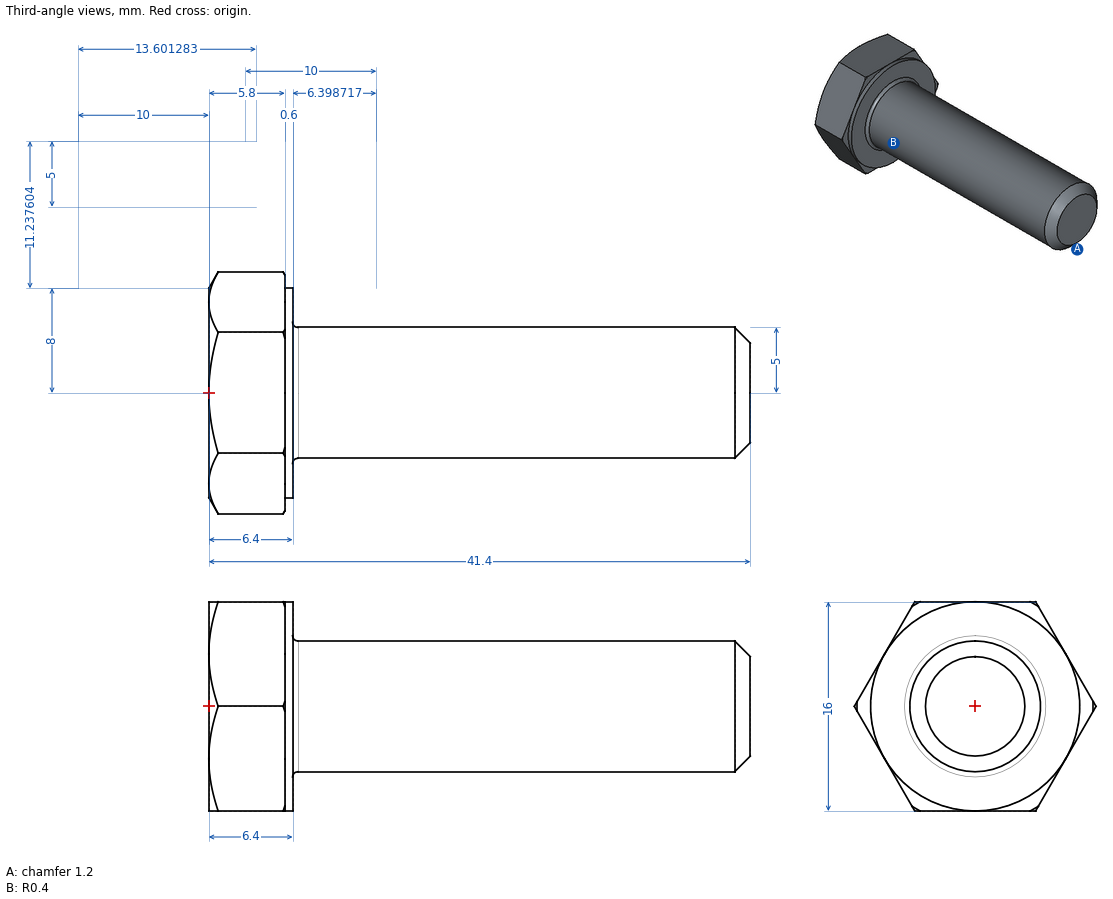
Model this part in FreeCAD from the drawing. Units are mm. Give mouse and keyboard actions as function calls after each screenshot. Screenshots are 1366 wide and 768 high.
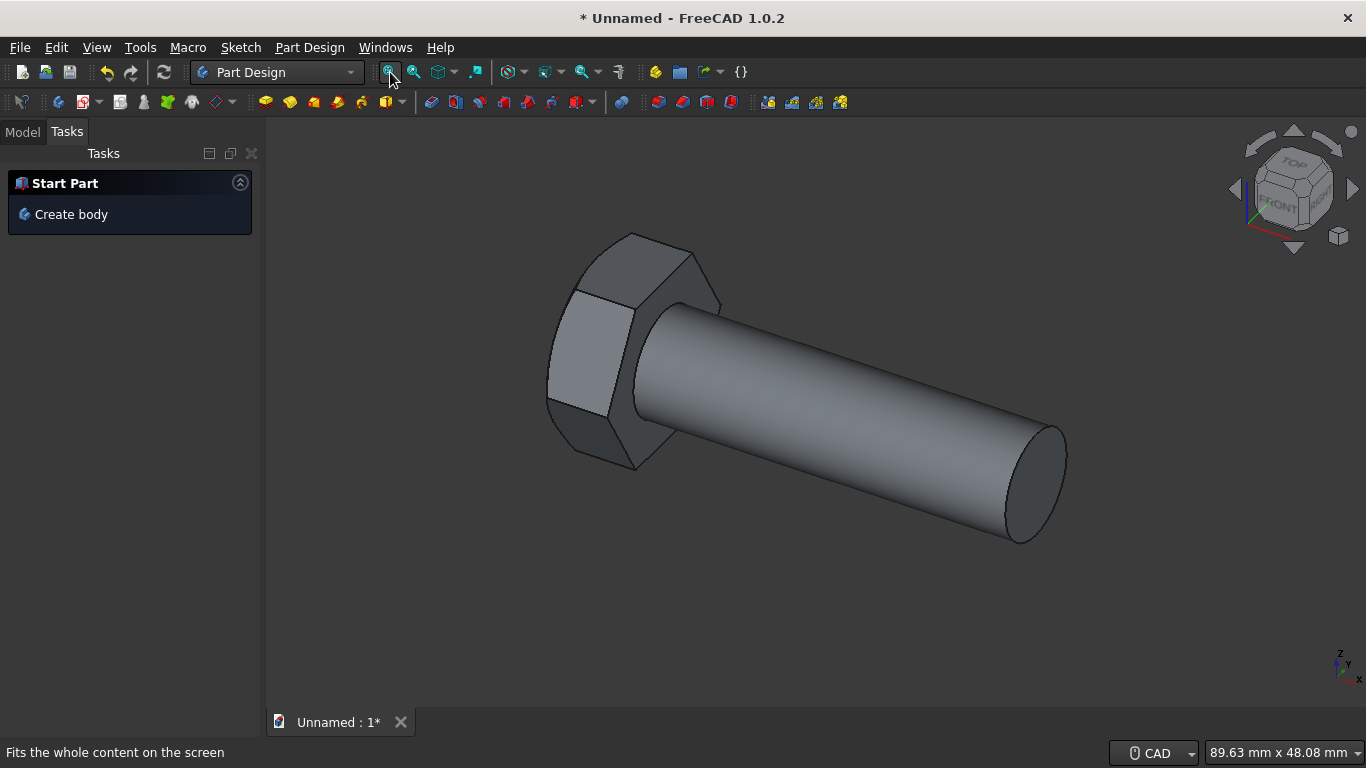
click(84, 102)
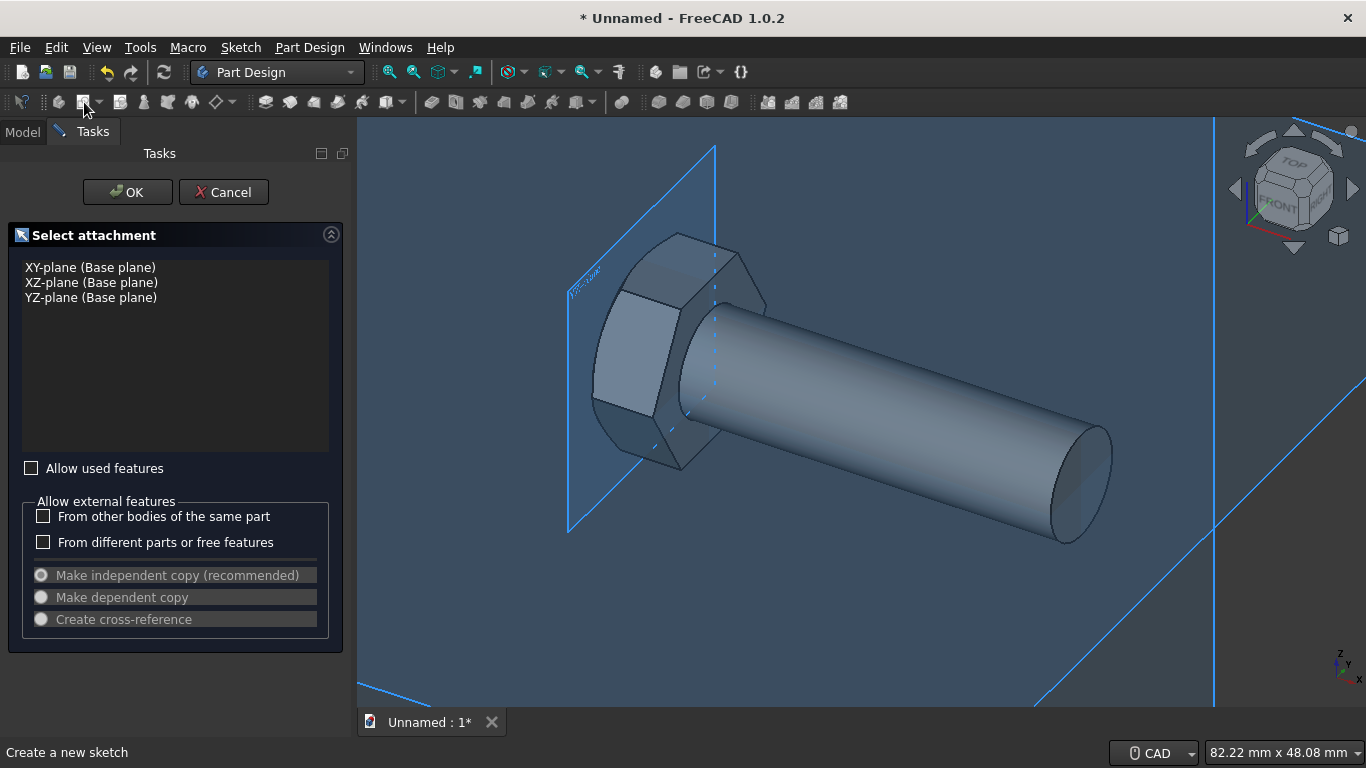
click(82, 268)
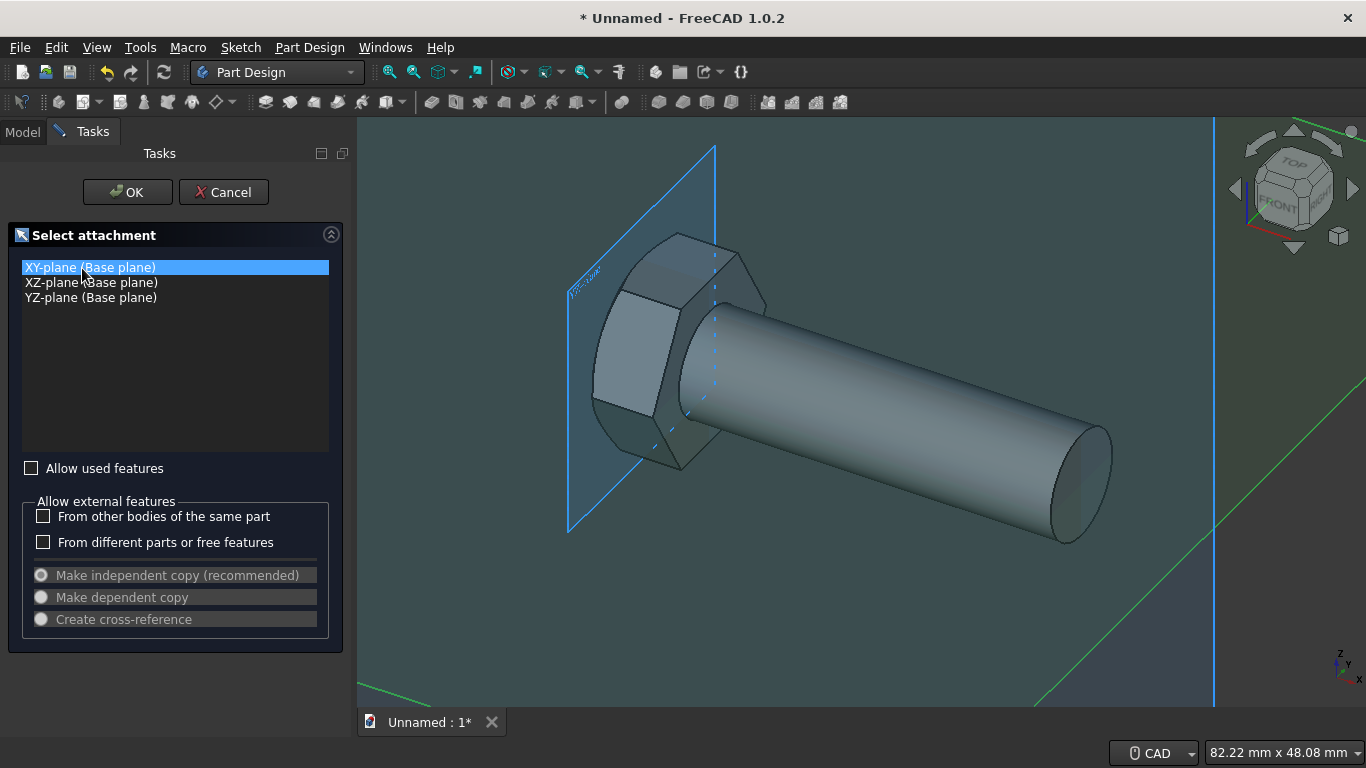
click(128, 192)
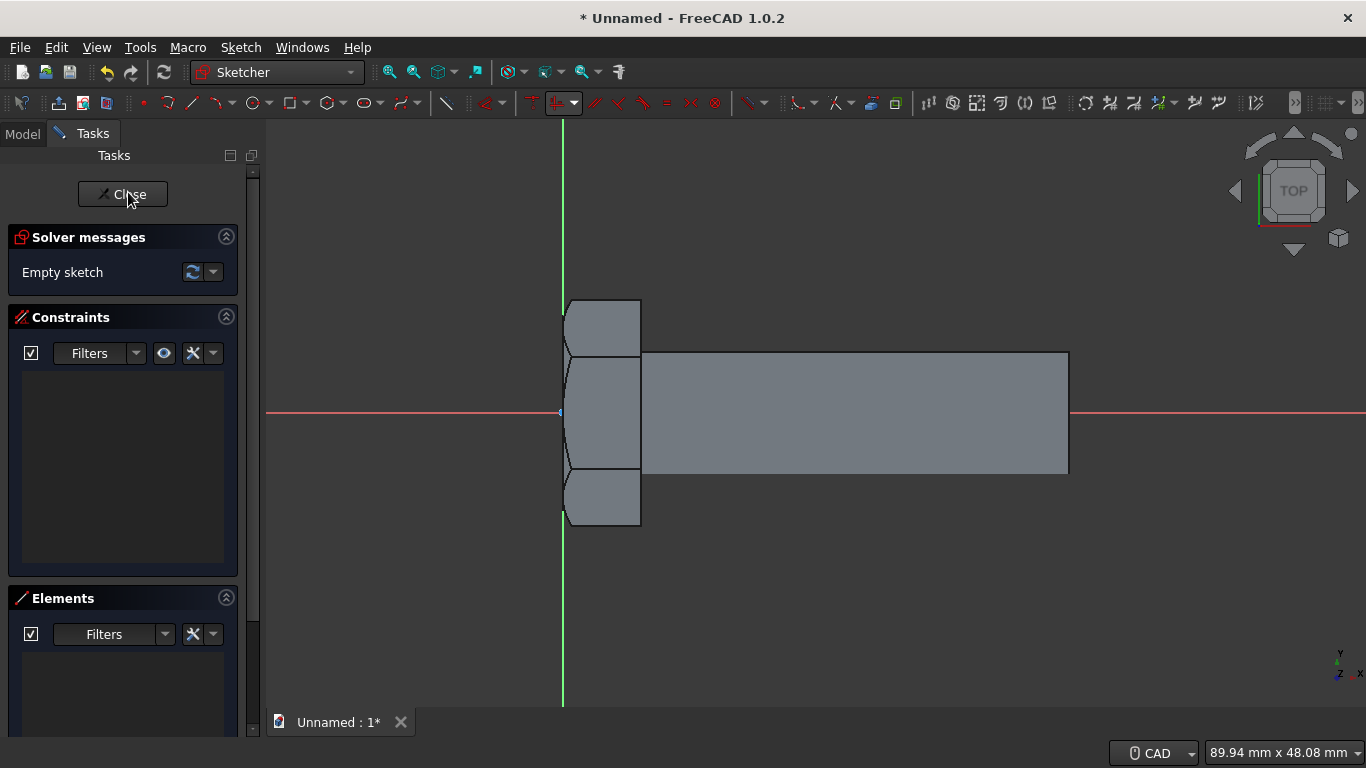
key(q)
key(s)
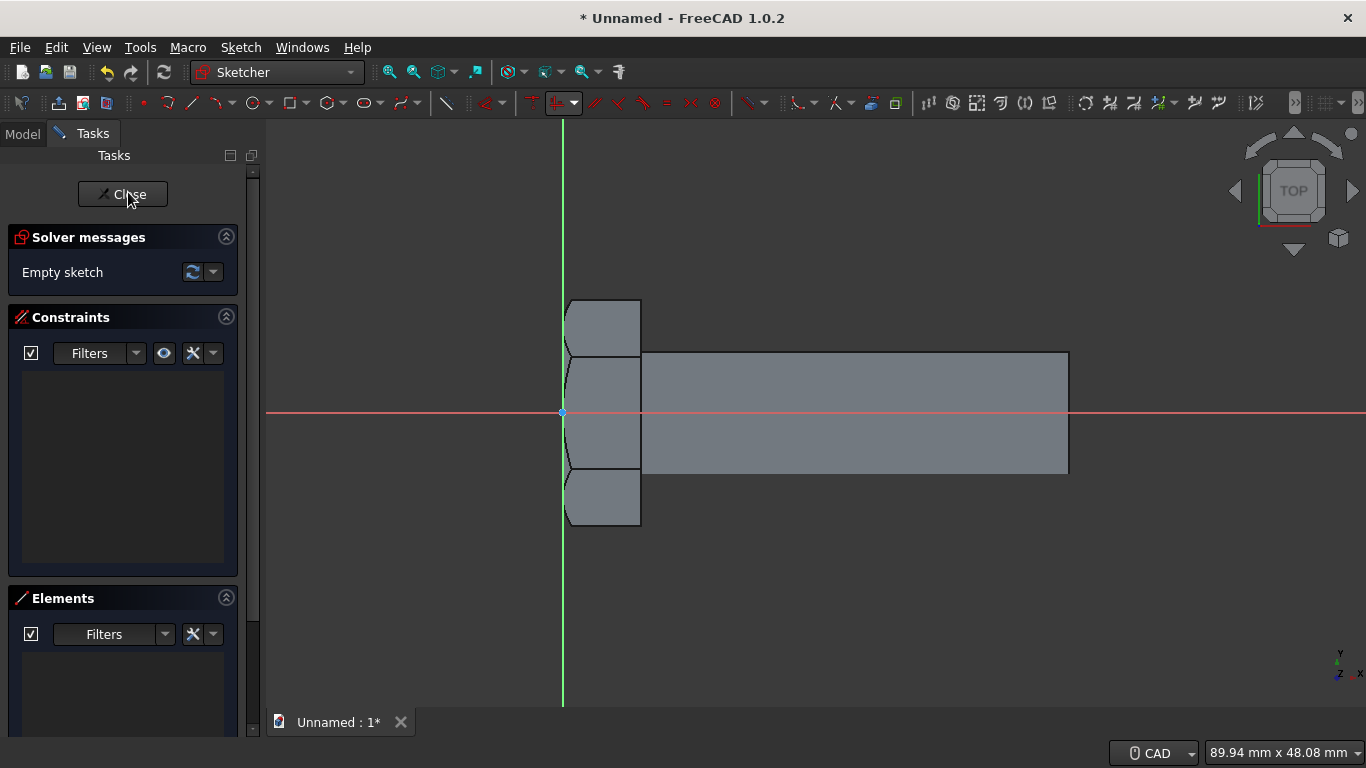
scroll(425, 147, up, 2)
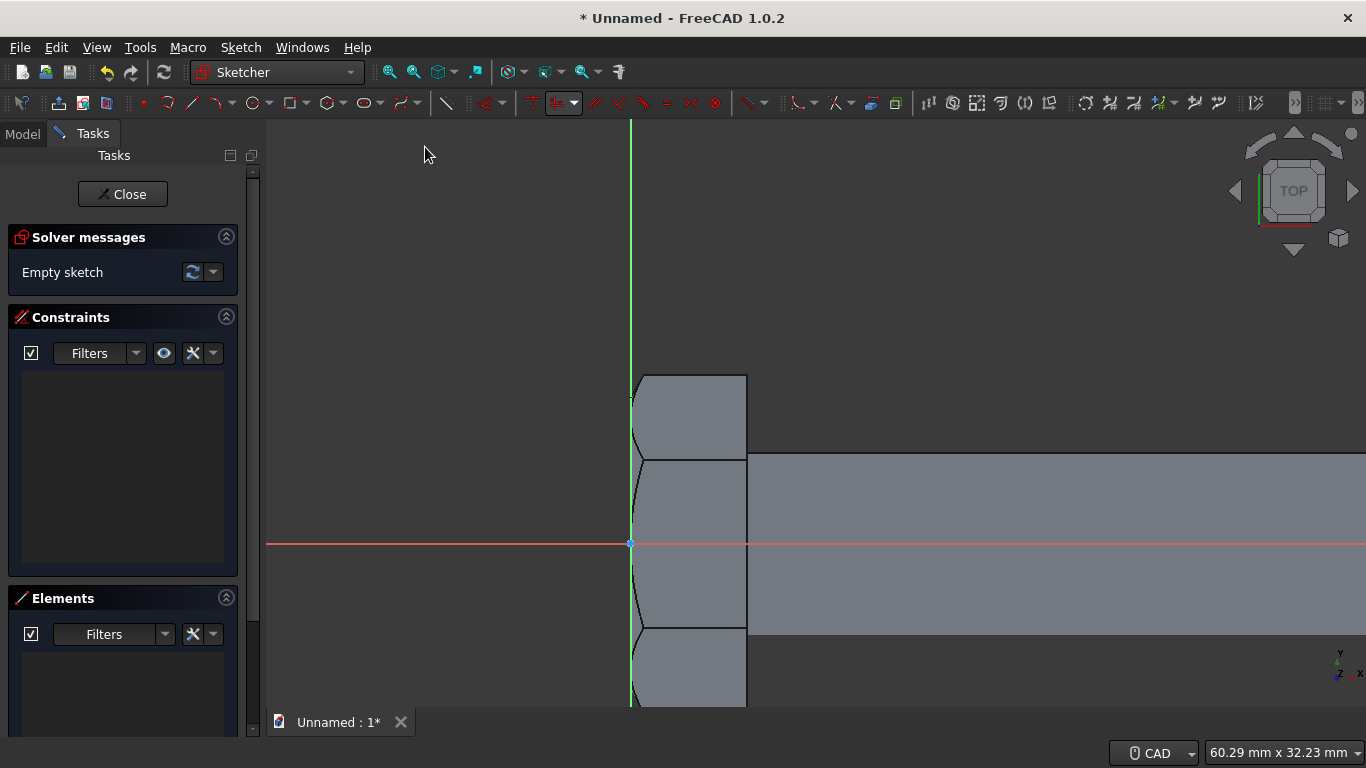
click(168, 104)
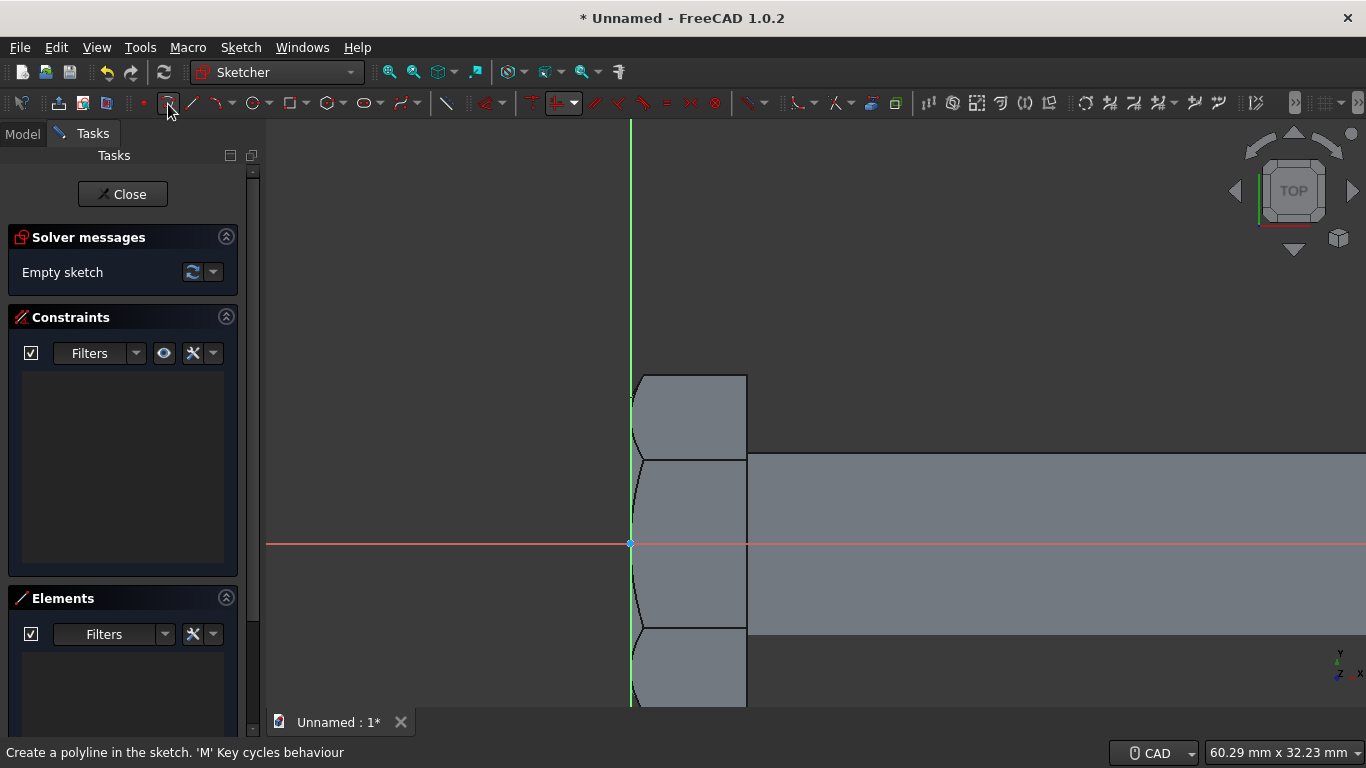
click(747, 398)
click(864, 398)
click(864, 193)
click(682, 193)
click(682, 284)
click(747, 399)
key(Escape)
key(Escape)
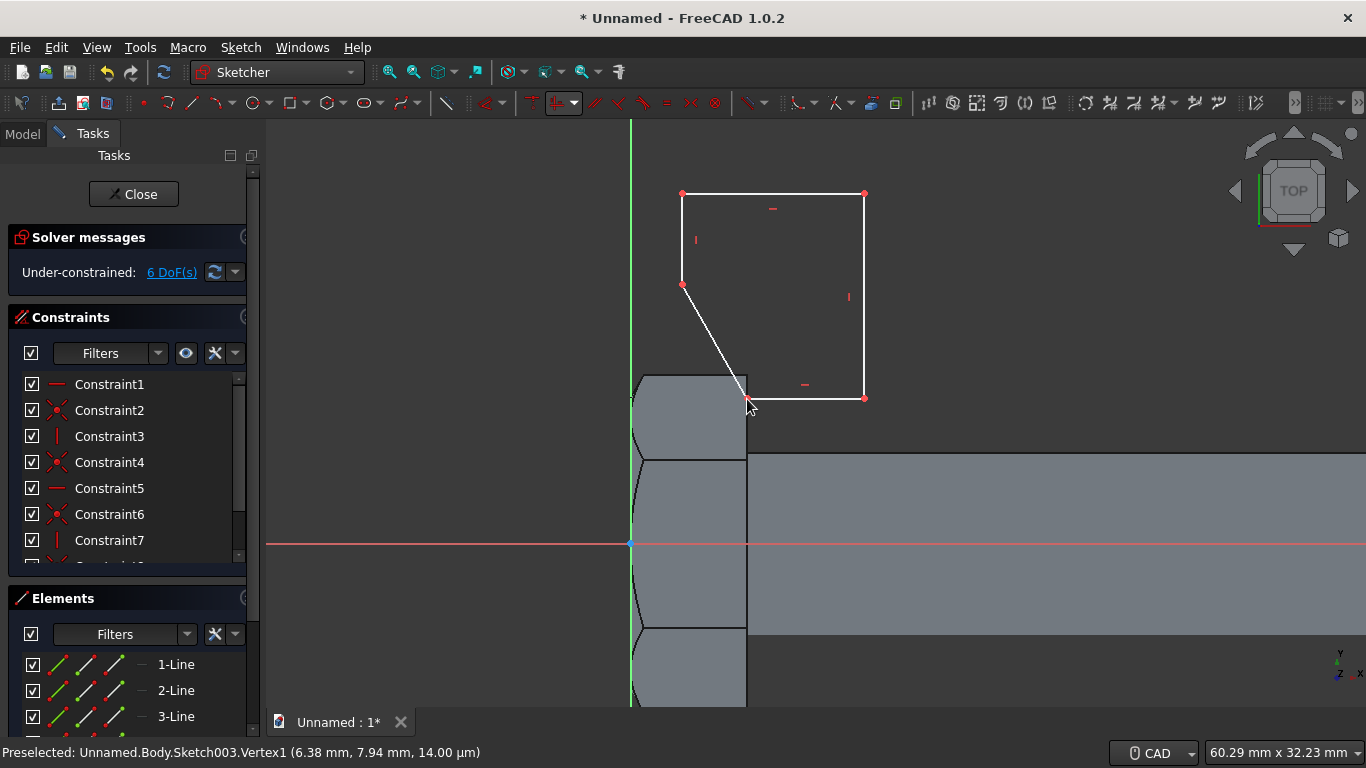
click(486, 104)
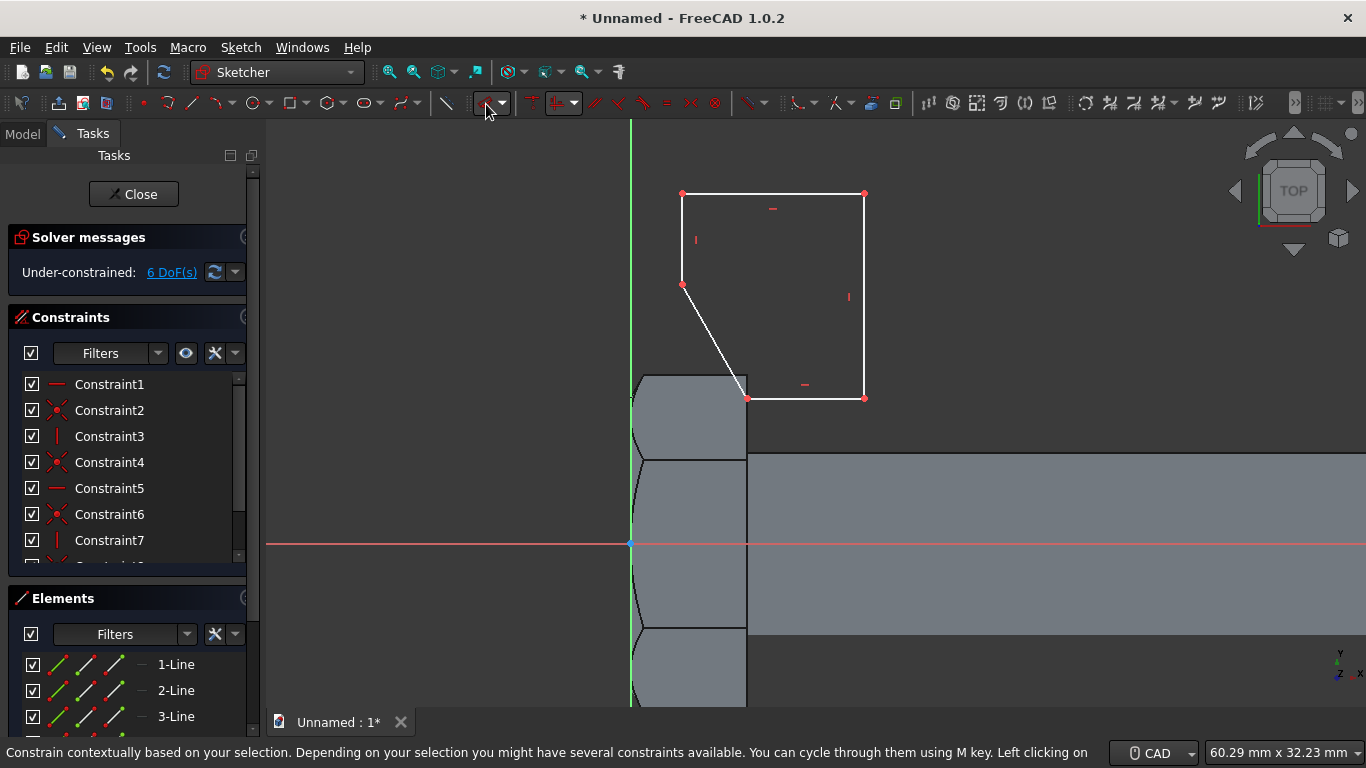
click(682, 221)
click(648, 240)